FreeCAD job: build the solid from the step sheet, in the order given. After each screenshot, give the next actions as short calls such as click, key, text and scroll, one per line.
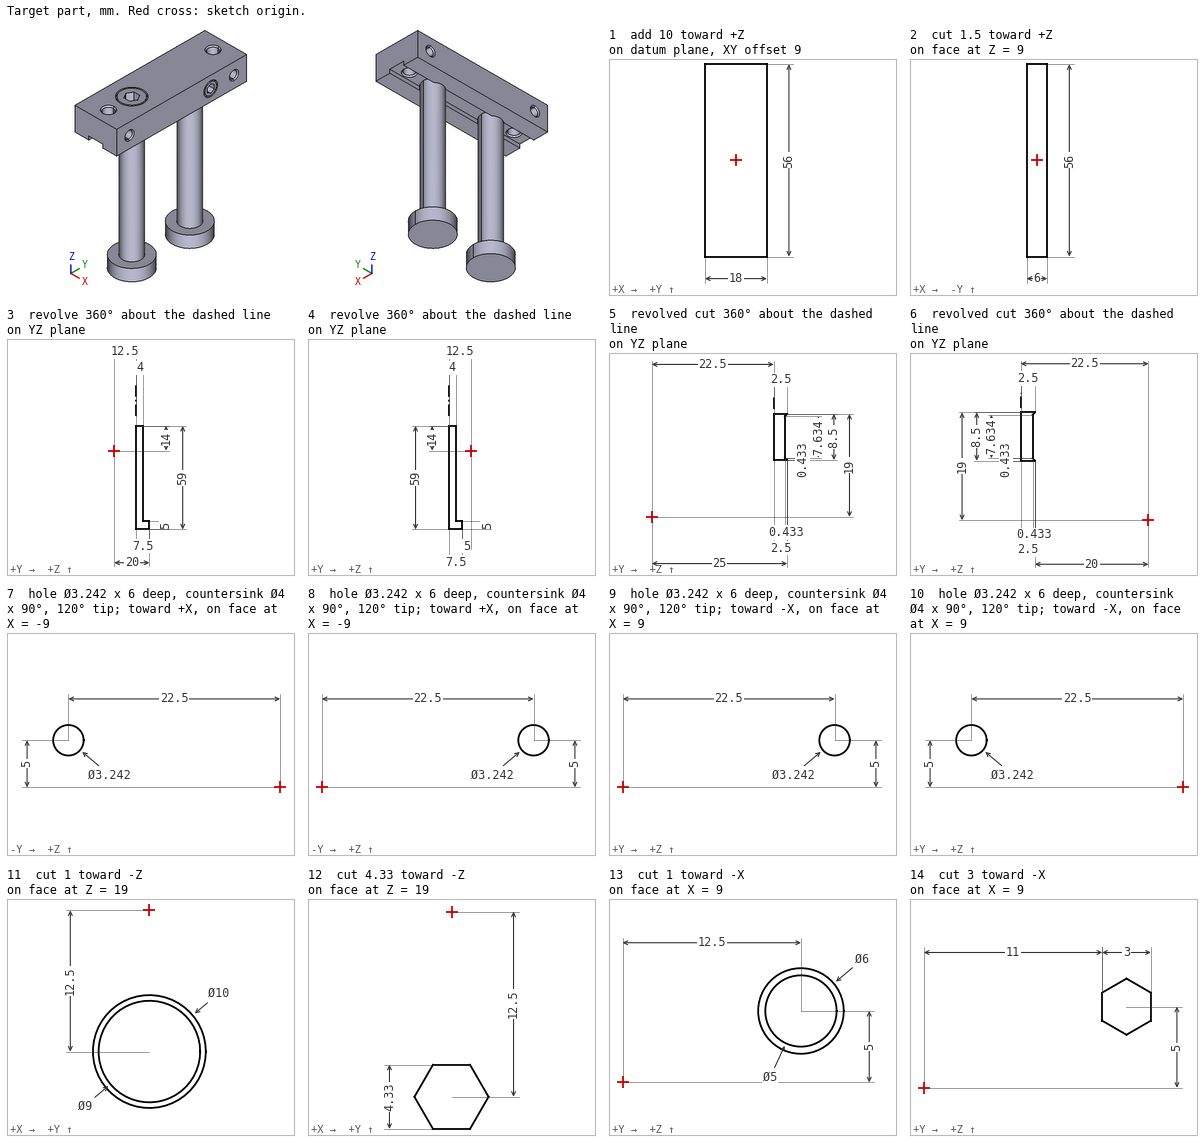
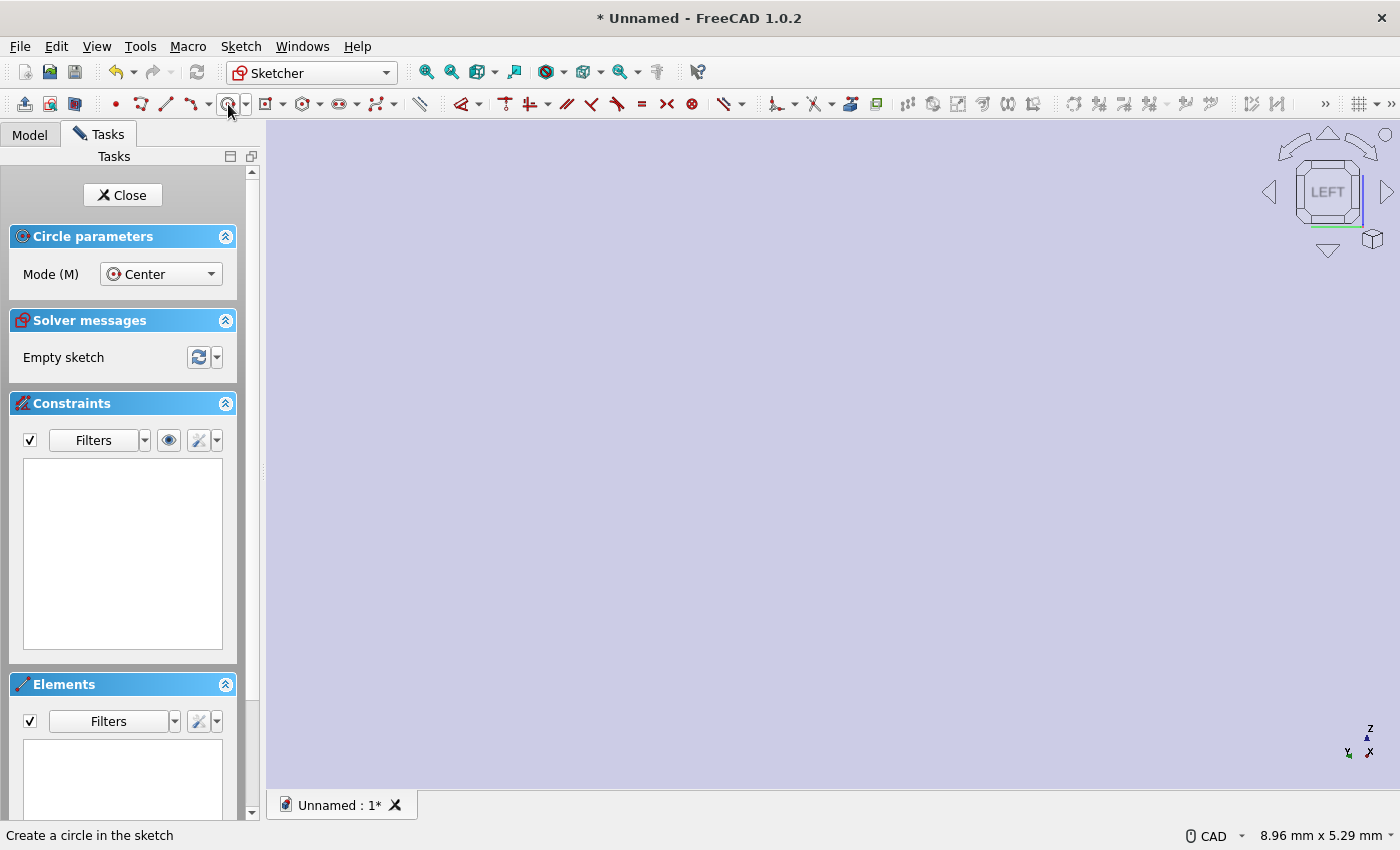
click(751, 456)
move(896, 311)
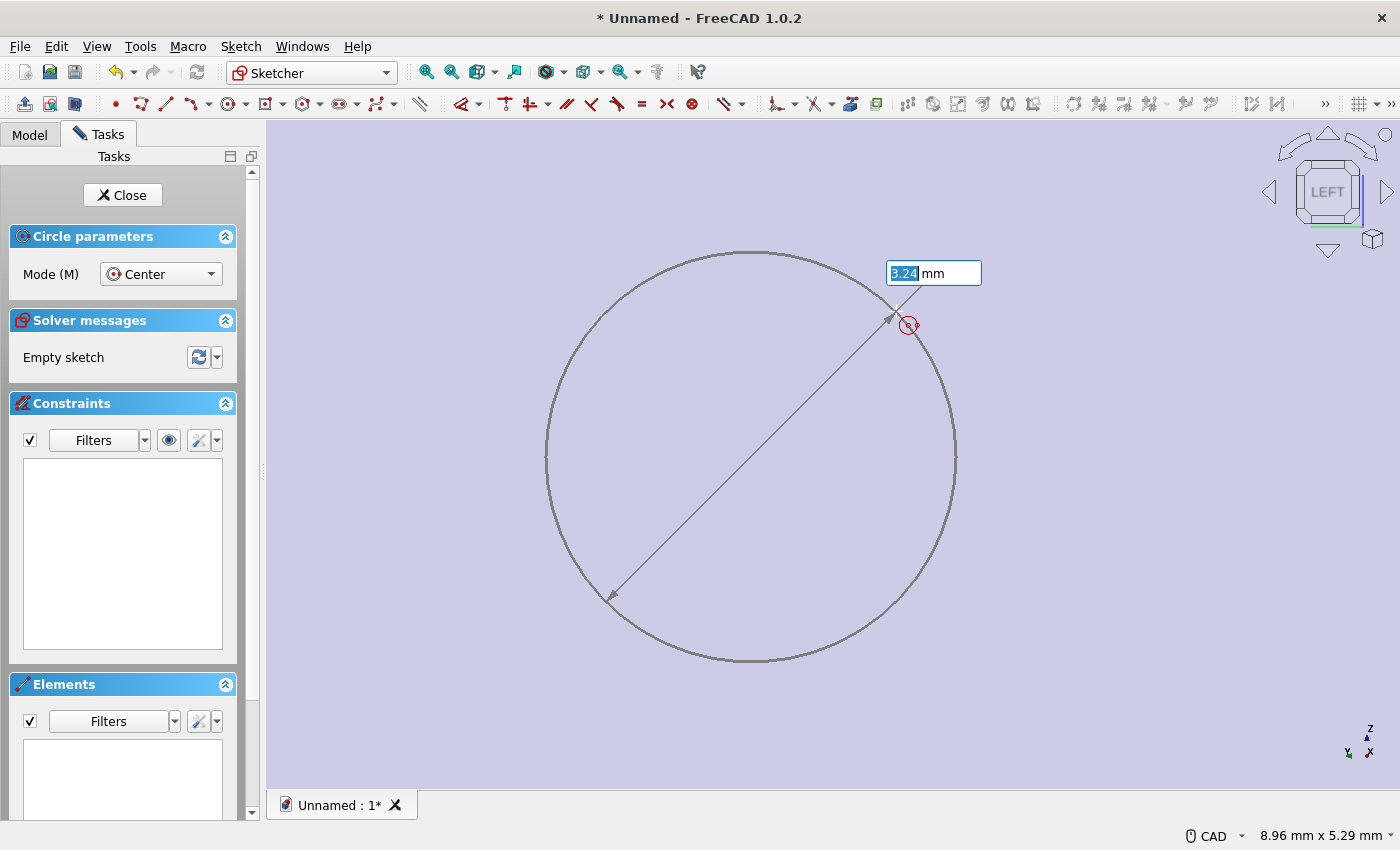
text(3.242)
key(Return)
key(Escape)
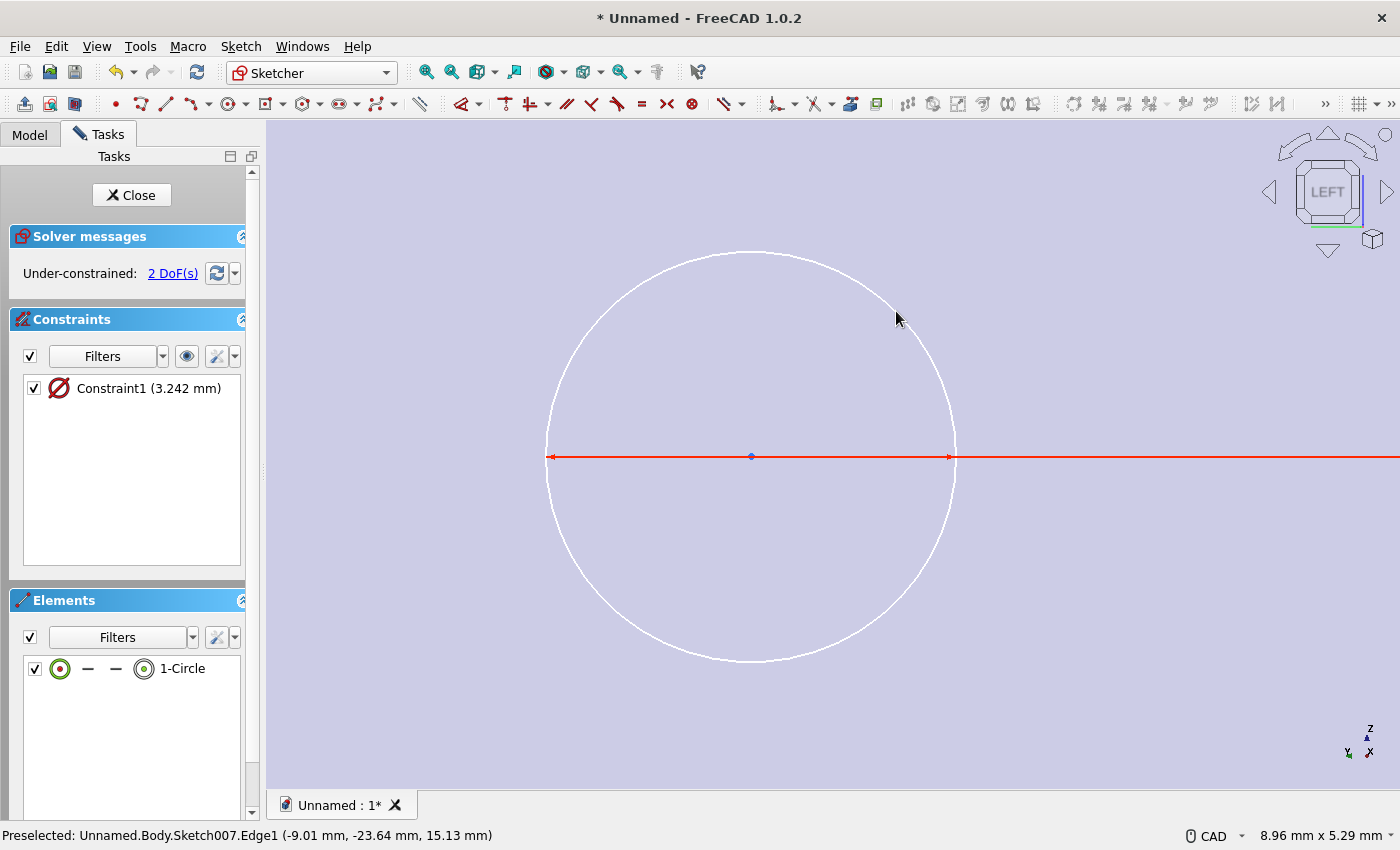
click(460, 104)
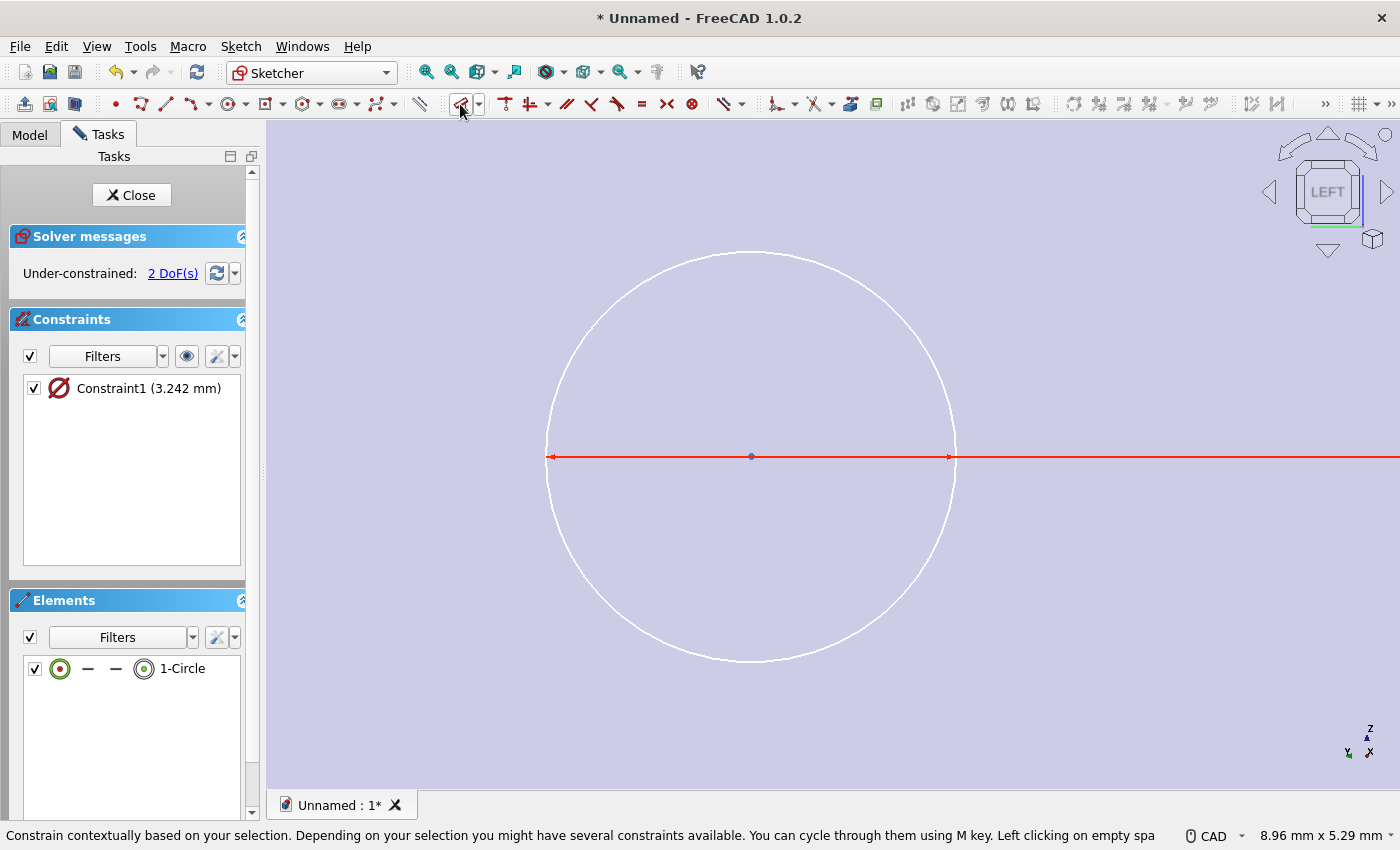
click(751, 457)
click(785, 609)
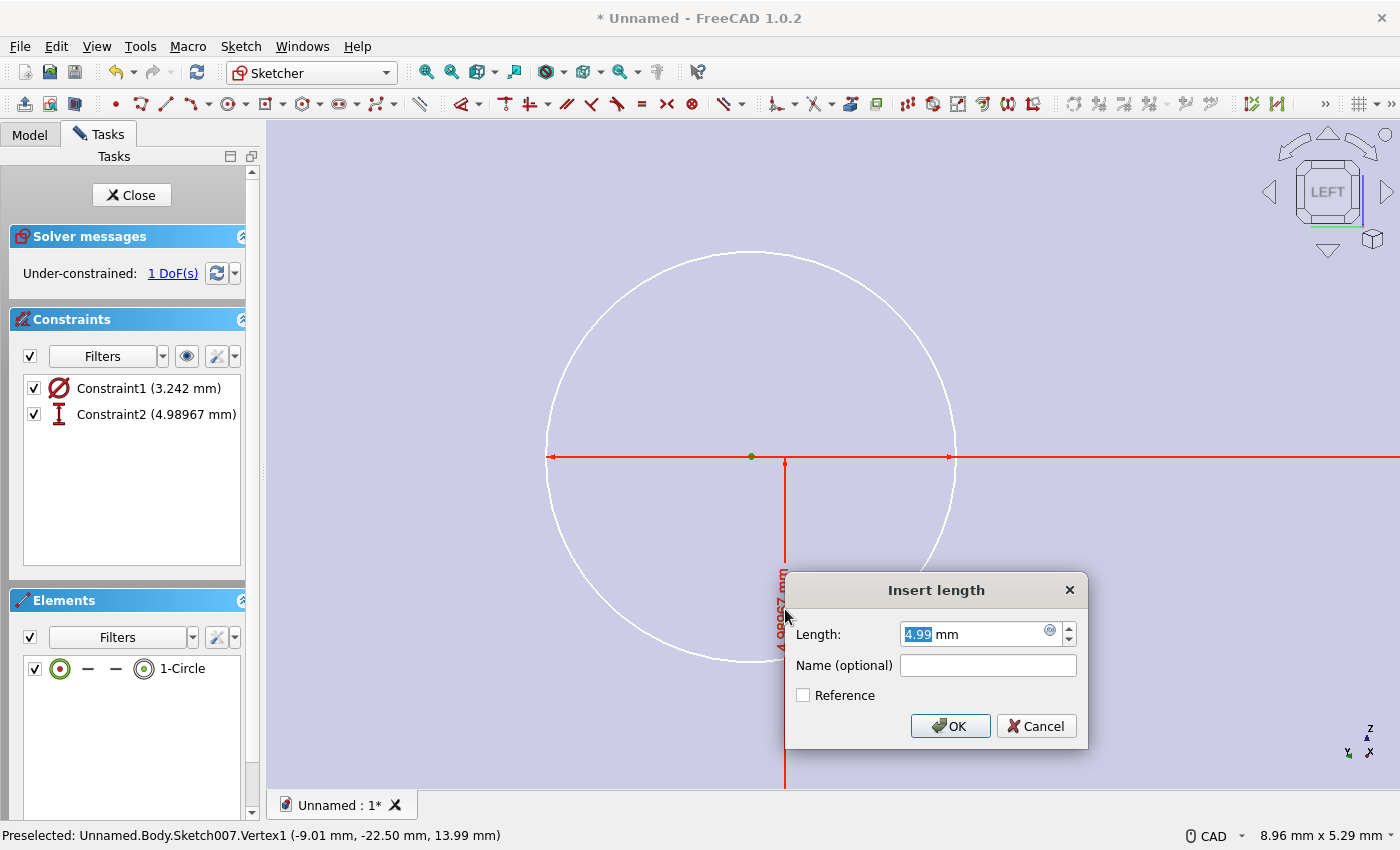
text(5)
key(Return)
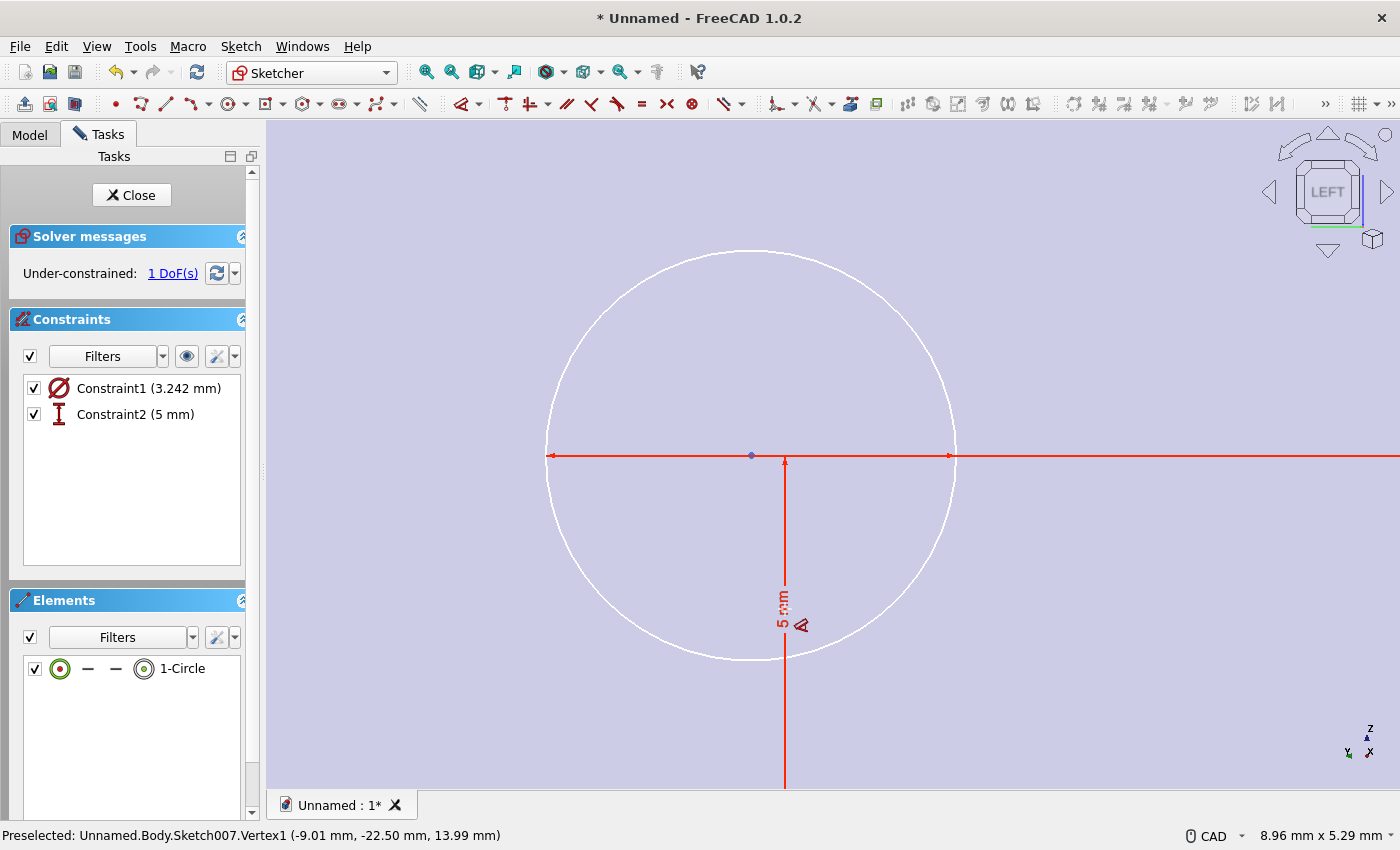
click(751, 456)
click(523, 422)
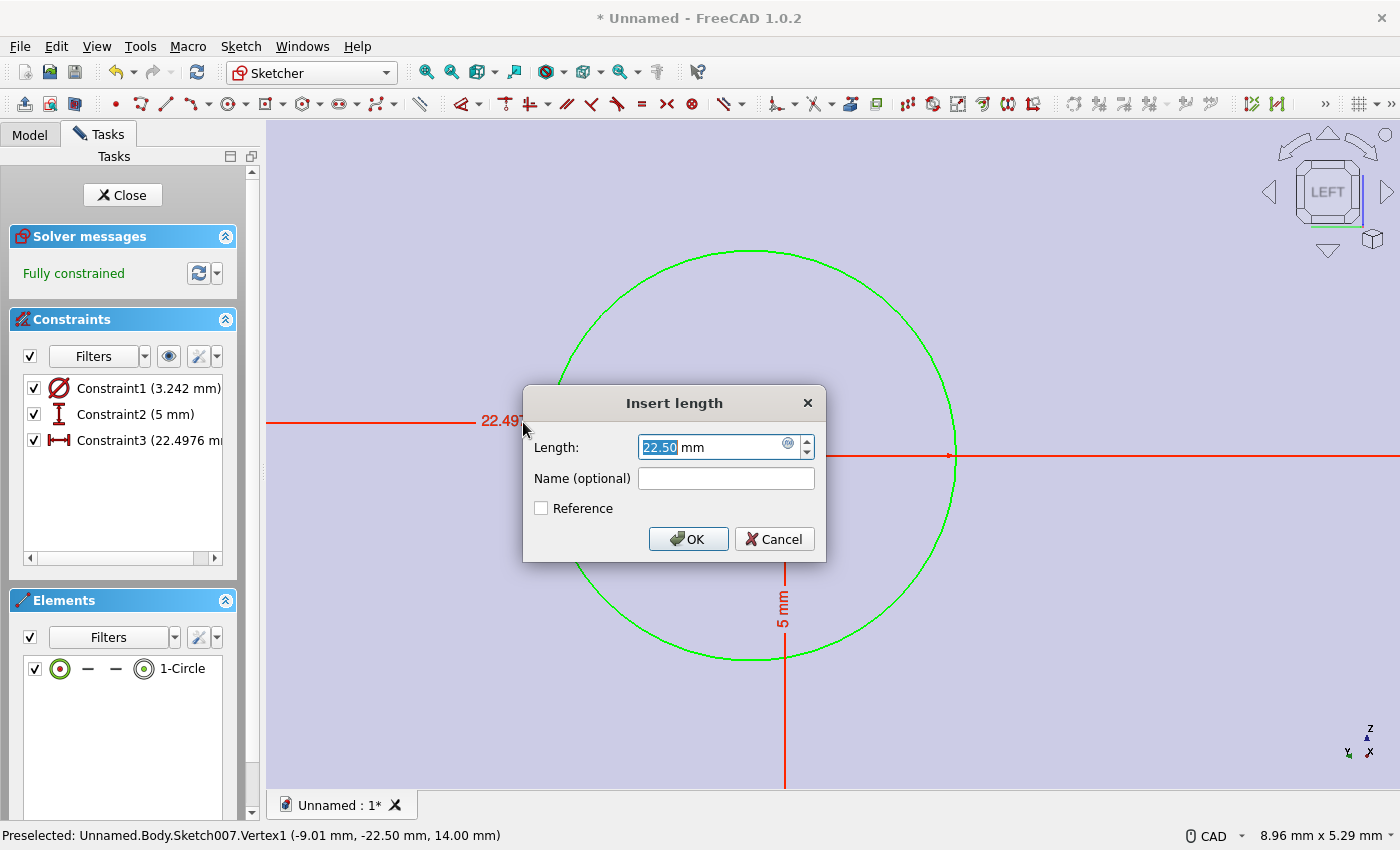
text(22.5)
key(Return)
key(Escape)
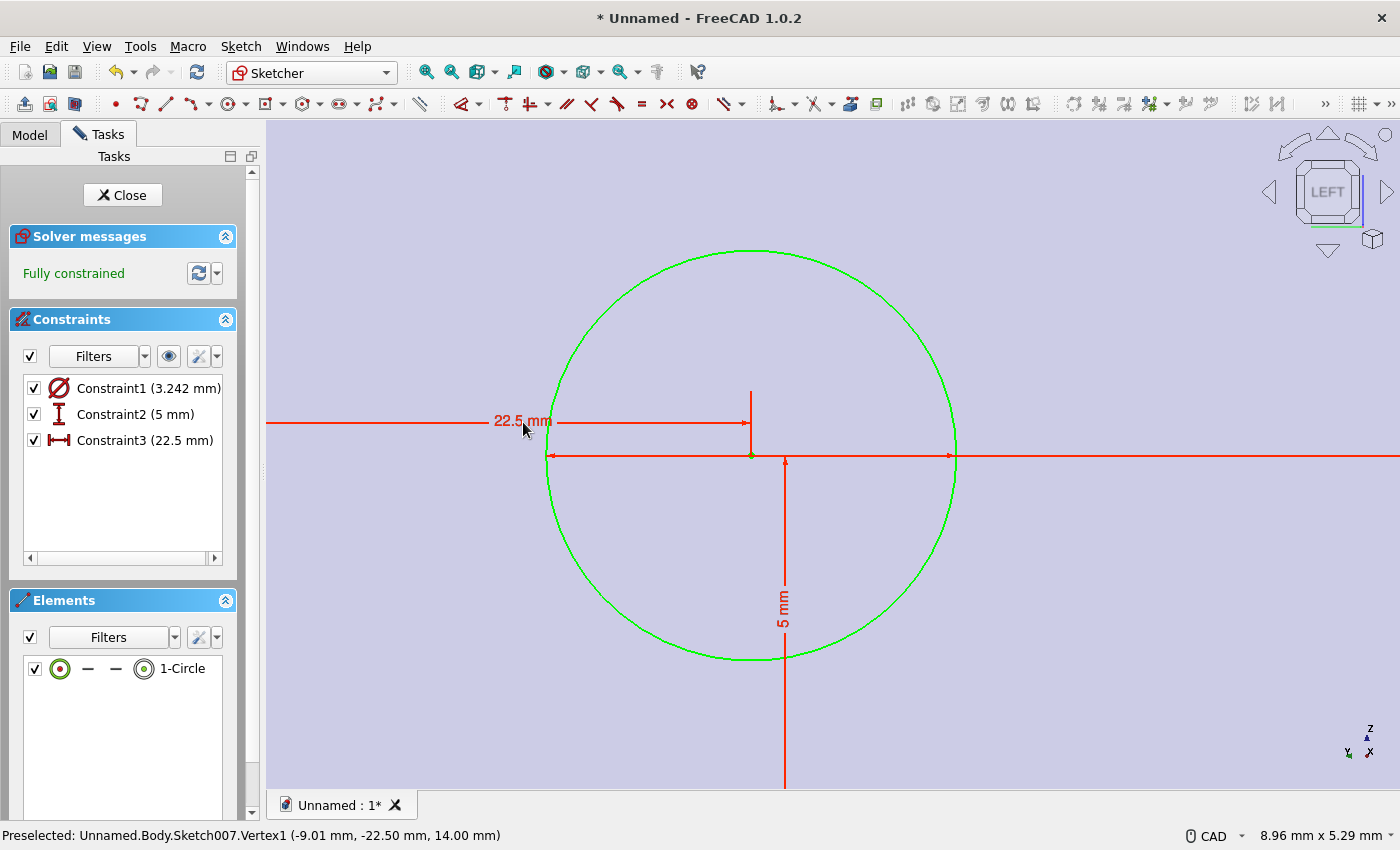
click(123, 195)